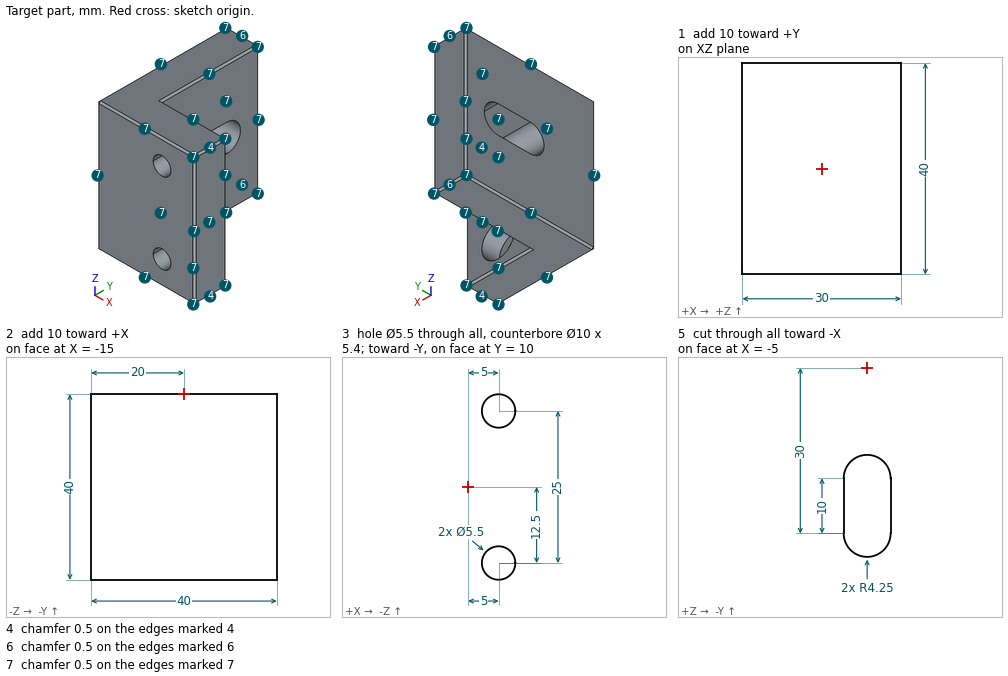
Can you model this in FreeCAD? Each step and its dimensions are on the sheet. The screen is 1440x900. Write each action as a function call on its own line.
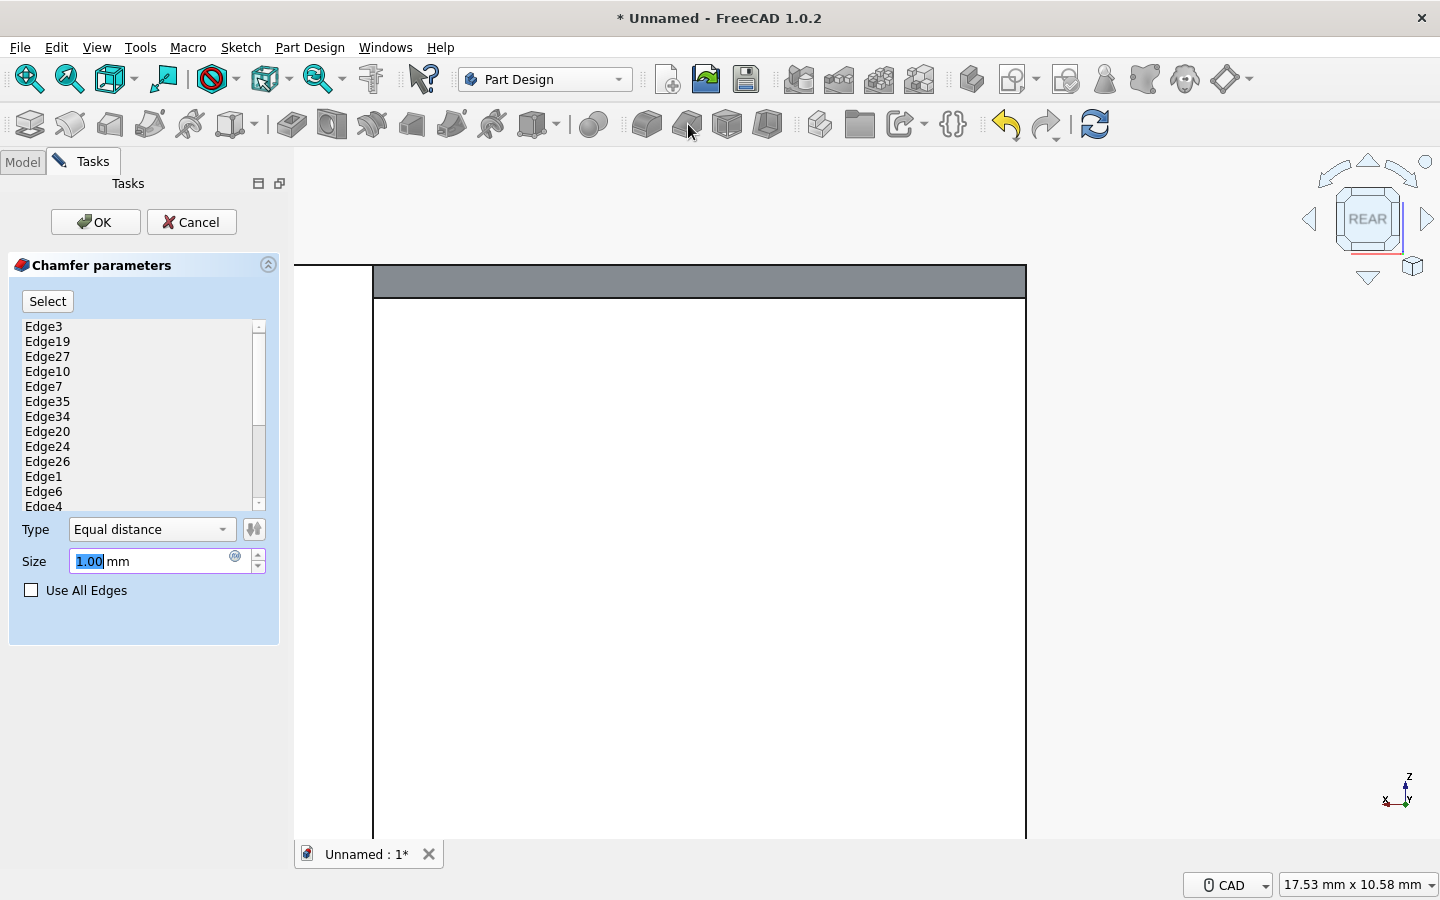
text(0.5)
key(Tab)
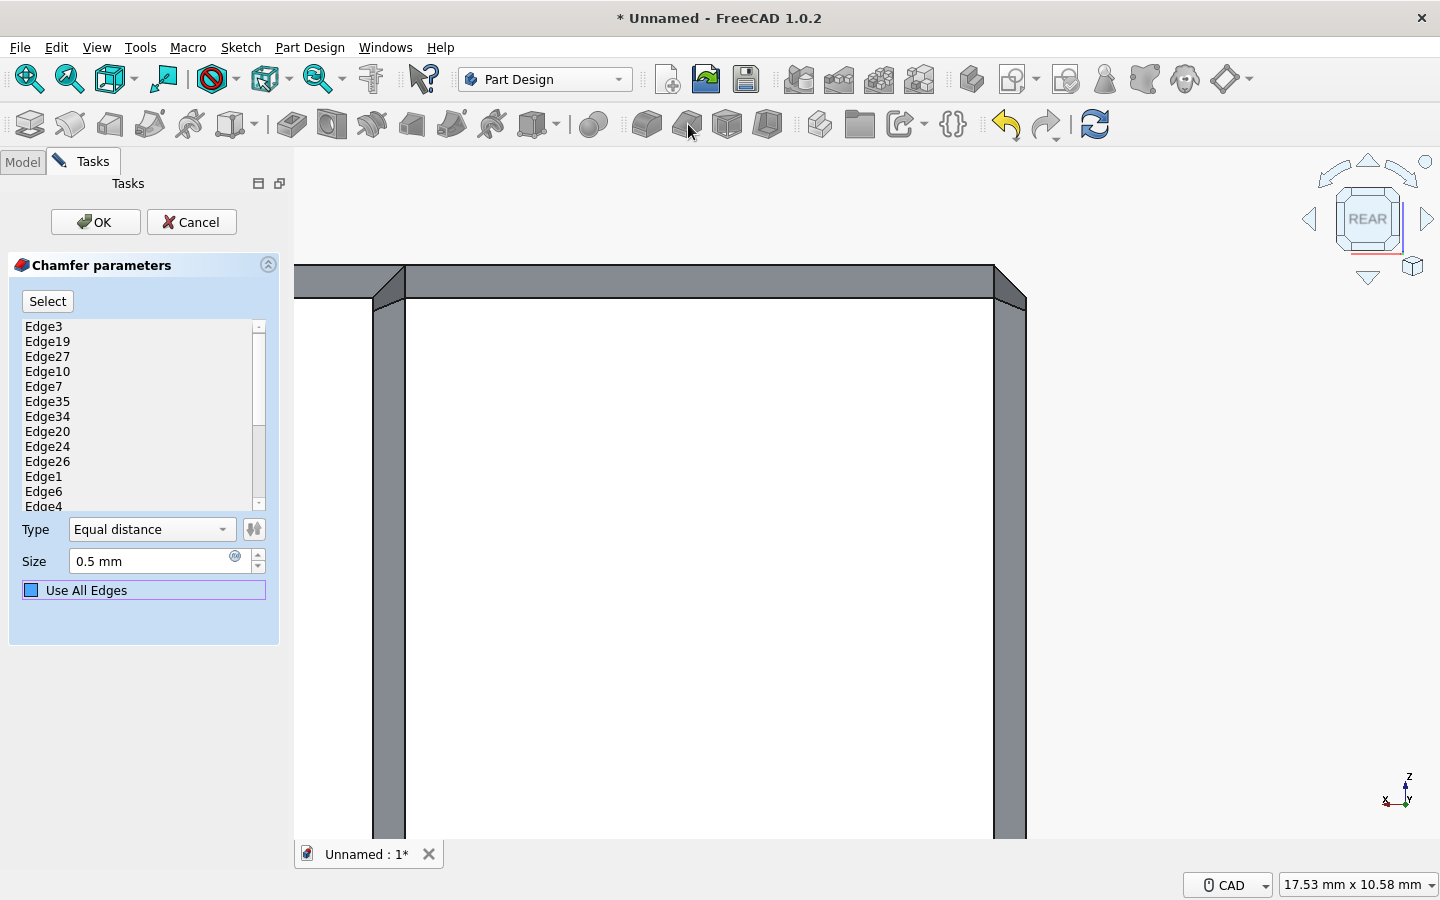
click(96, 222)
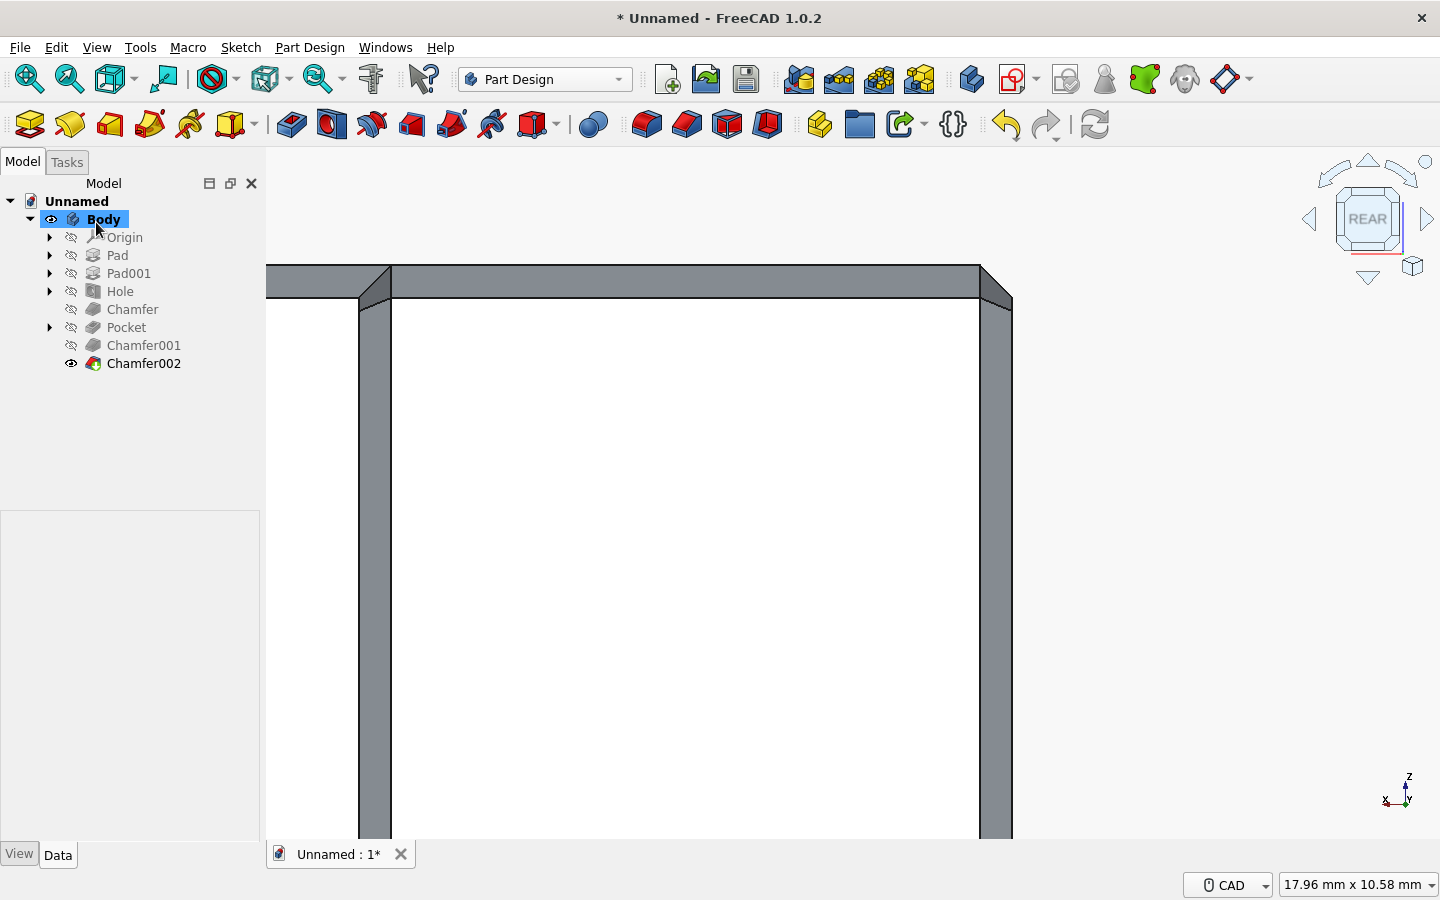
key(0)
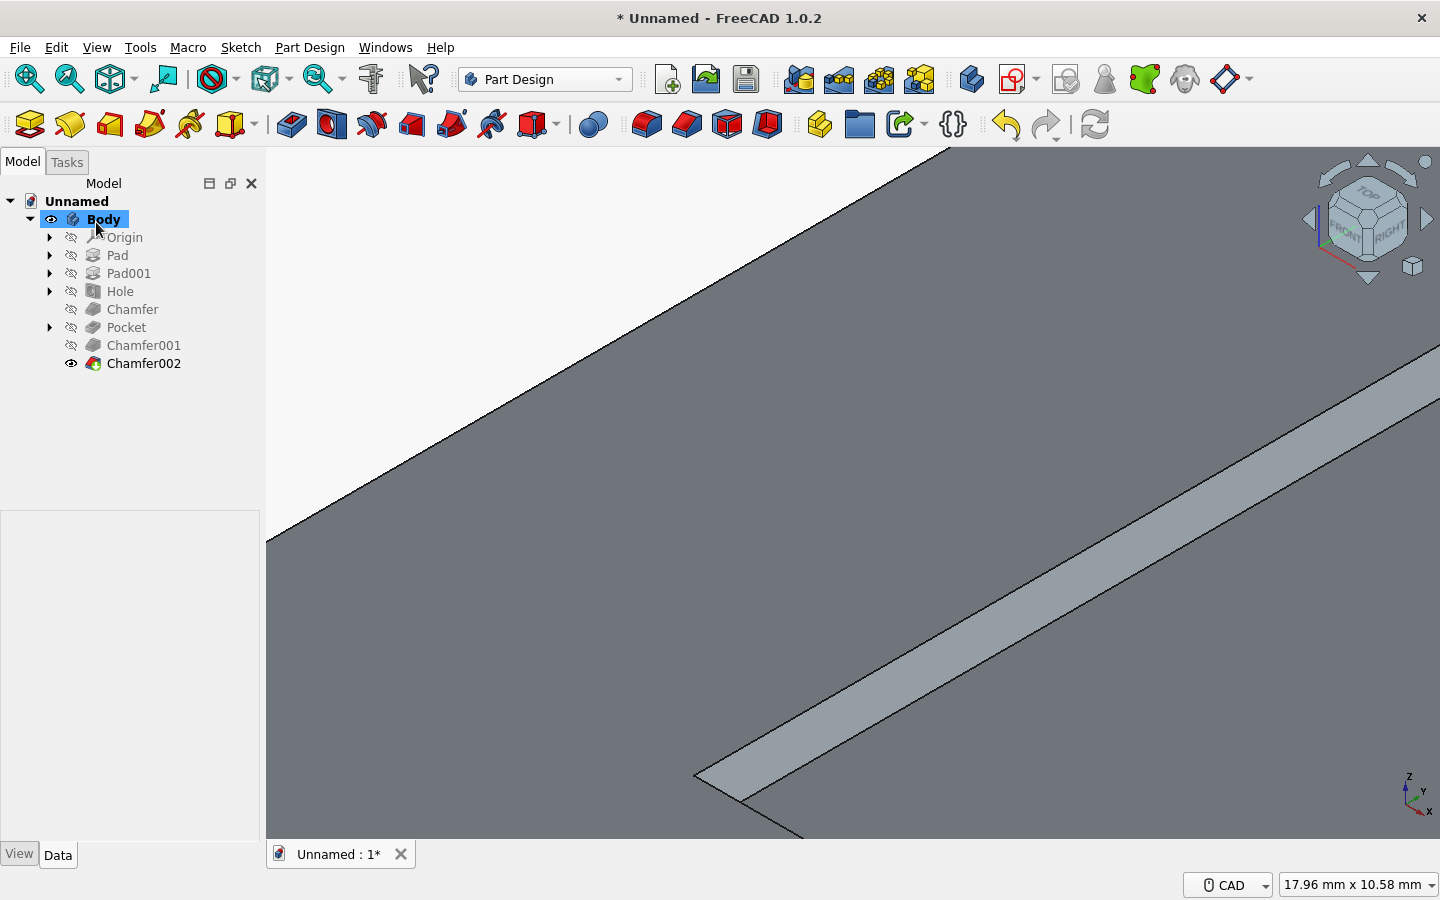
click(30, 80)